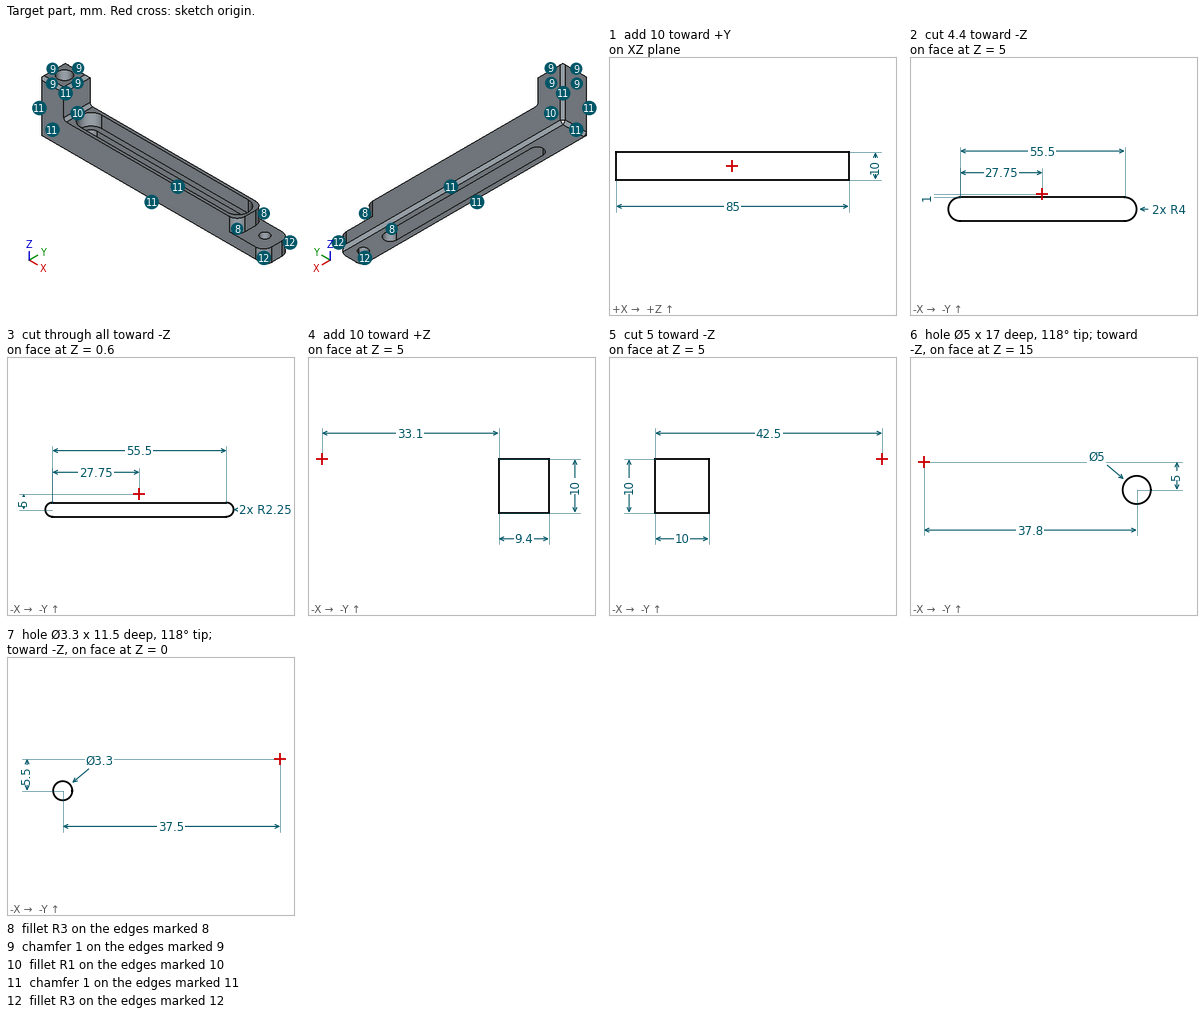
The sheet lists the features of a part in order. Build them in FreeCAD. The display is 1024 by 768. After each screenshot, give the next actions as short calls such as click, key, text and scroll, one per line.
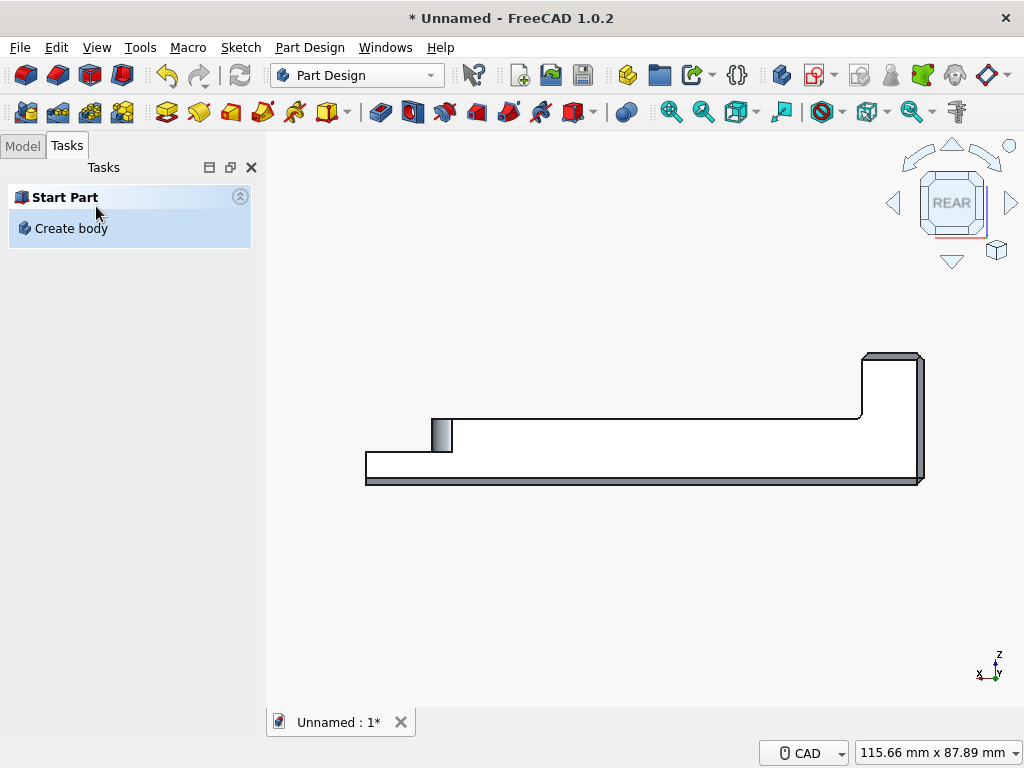
click(366, 464)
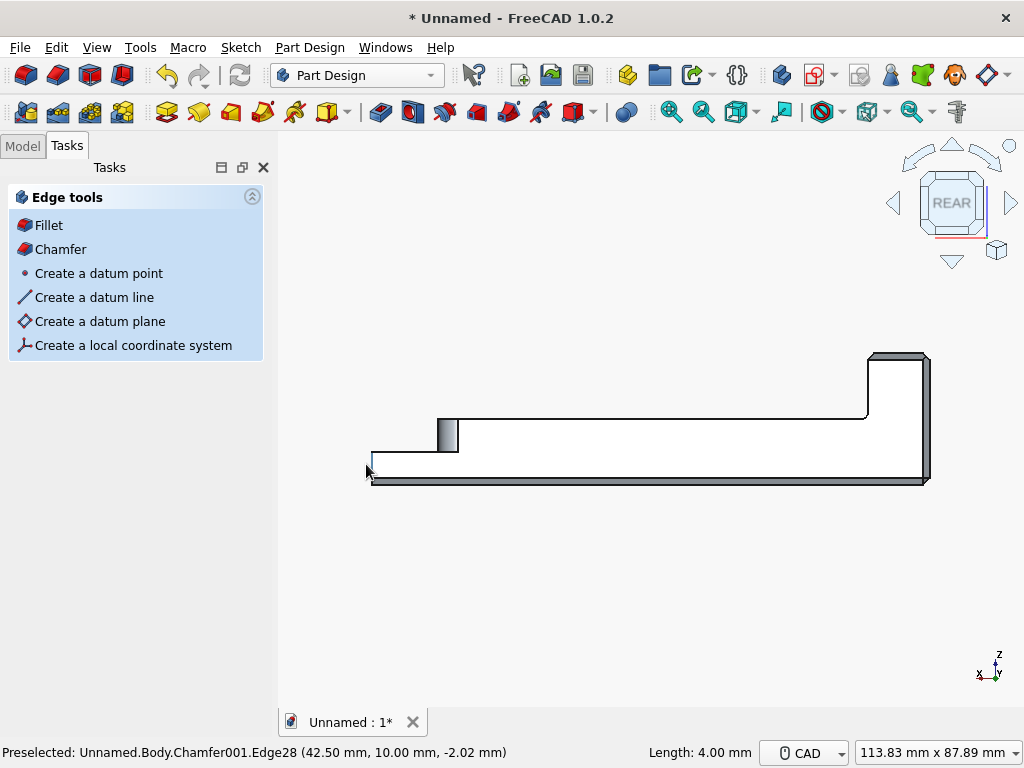
key(0)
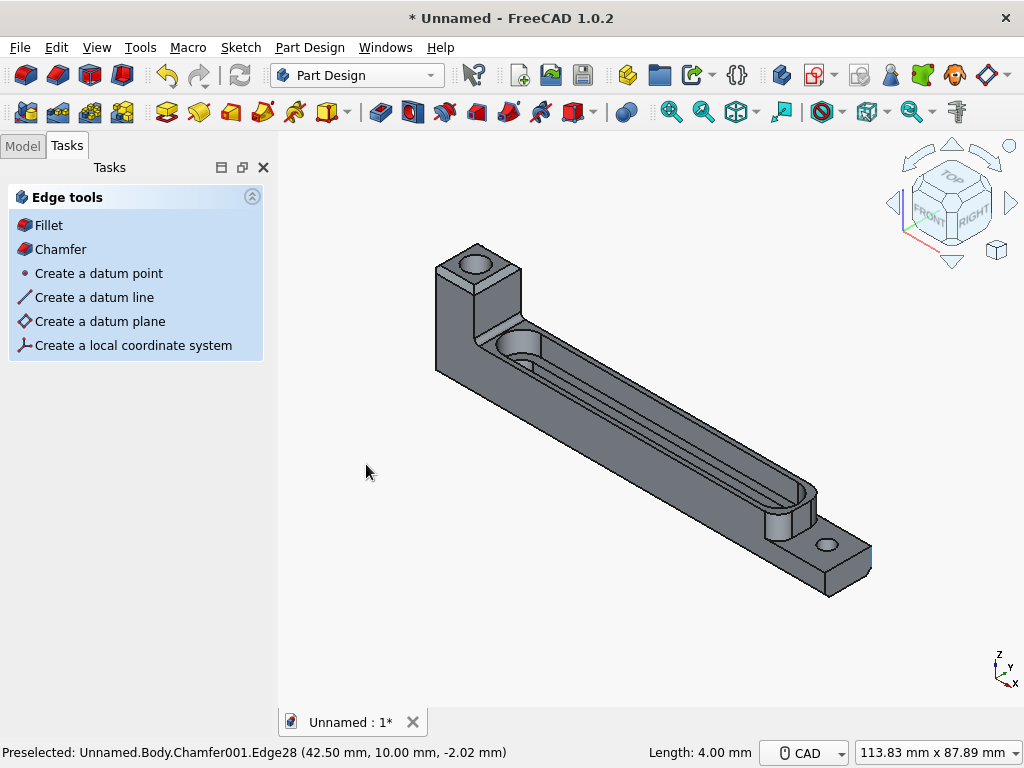
click(825, 583, ctrl)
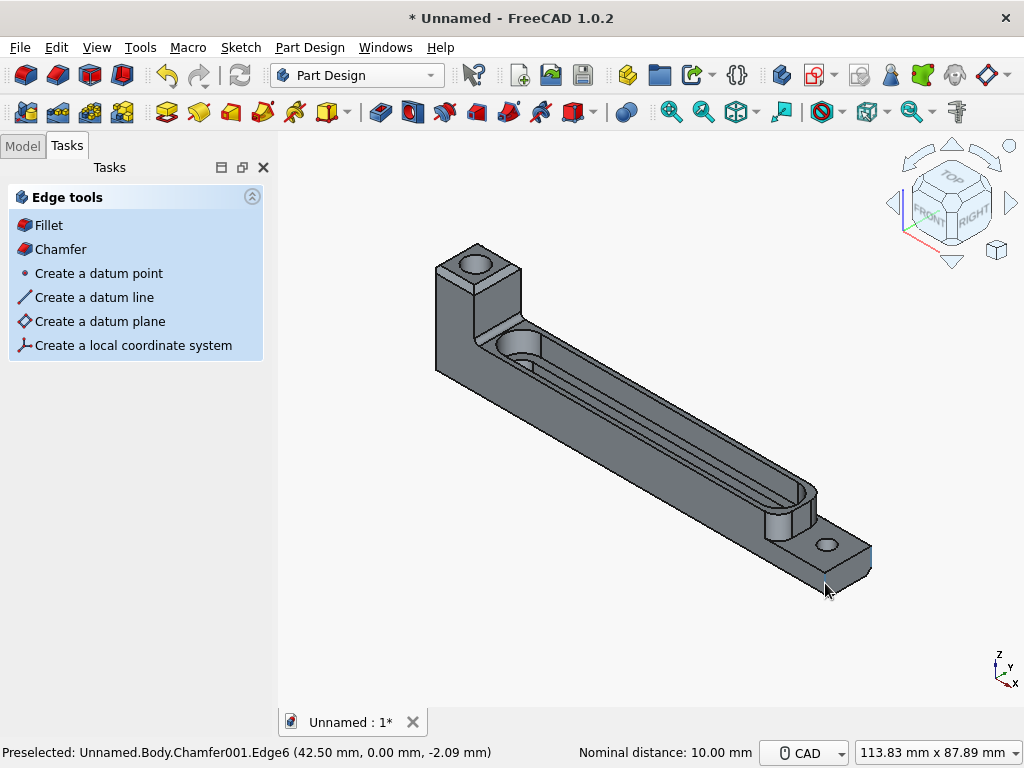
click(26, 76)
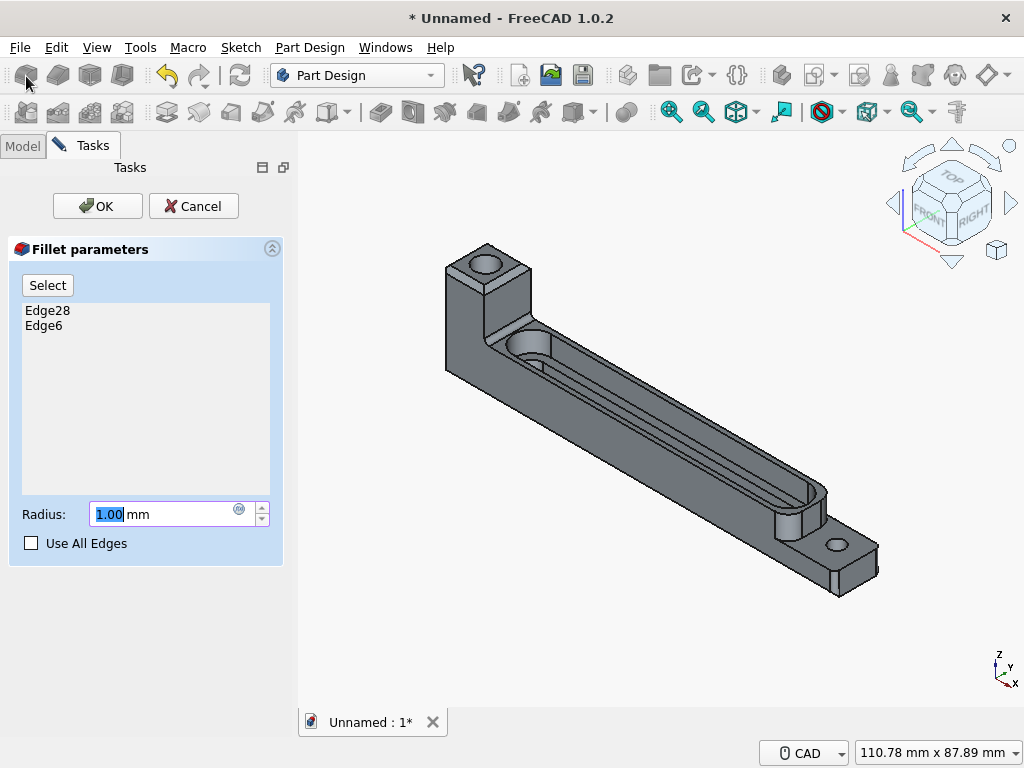
text(3)
key(Tab)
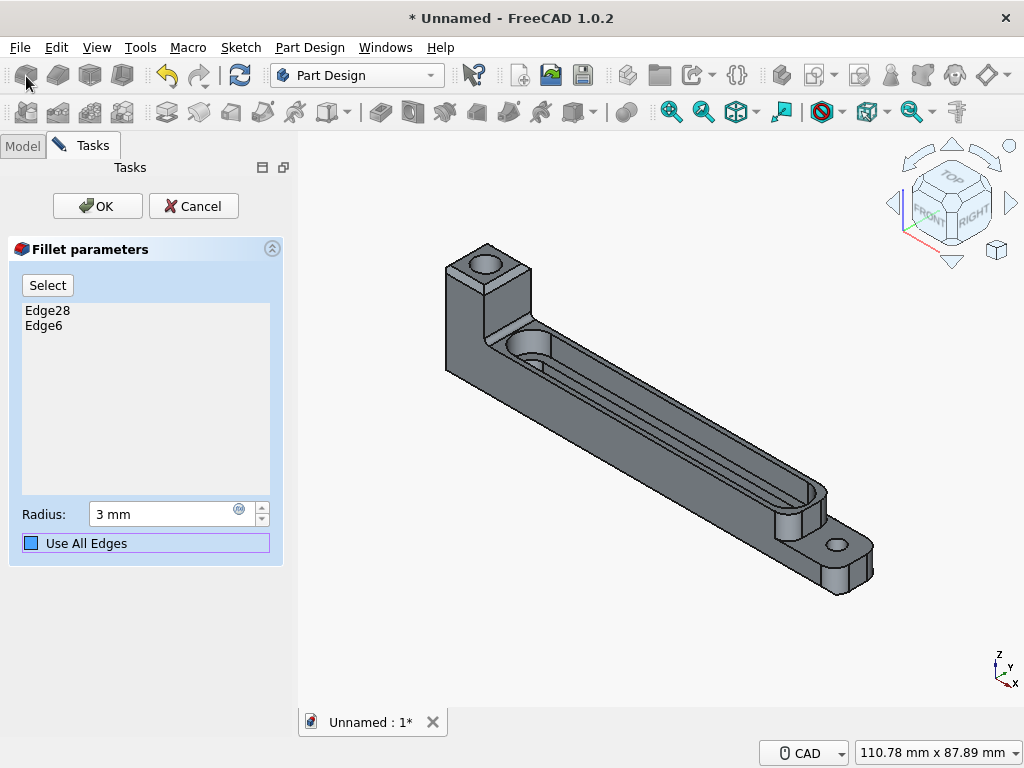
click(98, 206)